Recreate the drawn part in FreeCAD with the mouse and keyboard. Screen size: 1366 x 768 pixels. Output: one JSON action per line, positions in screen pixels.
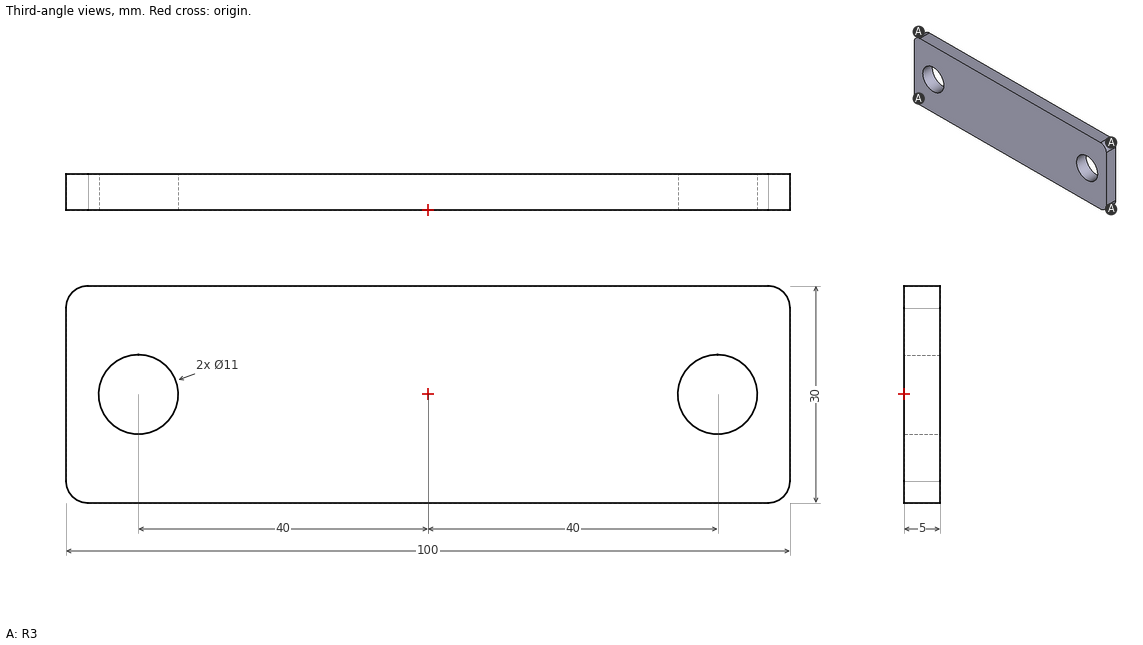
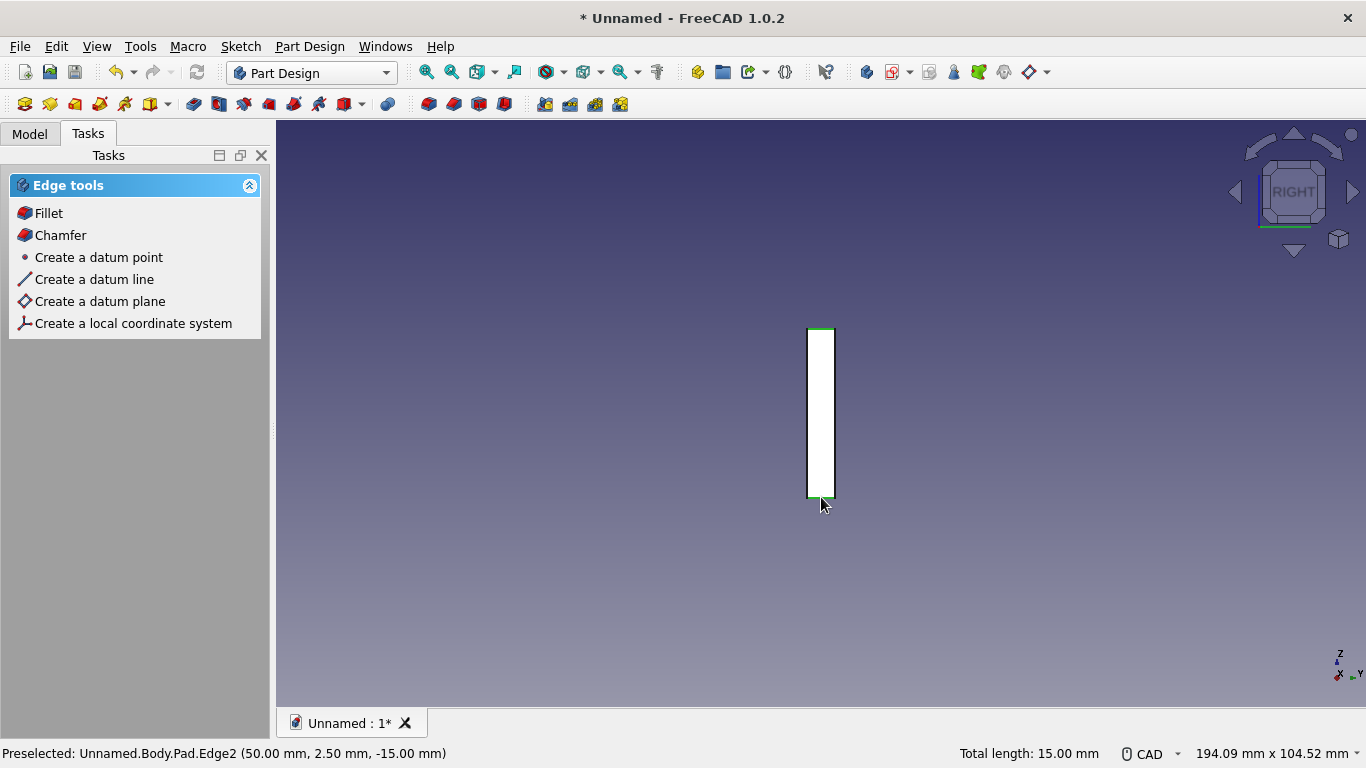
{"action": "key", "text": "5"}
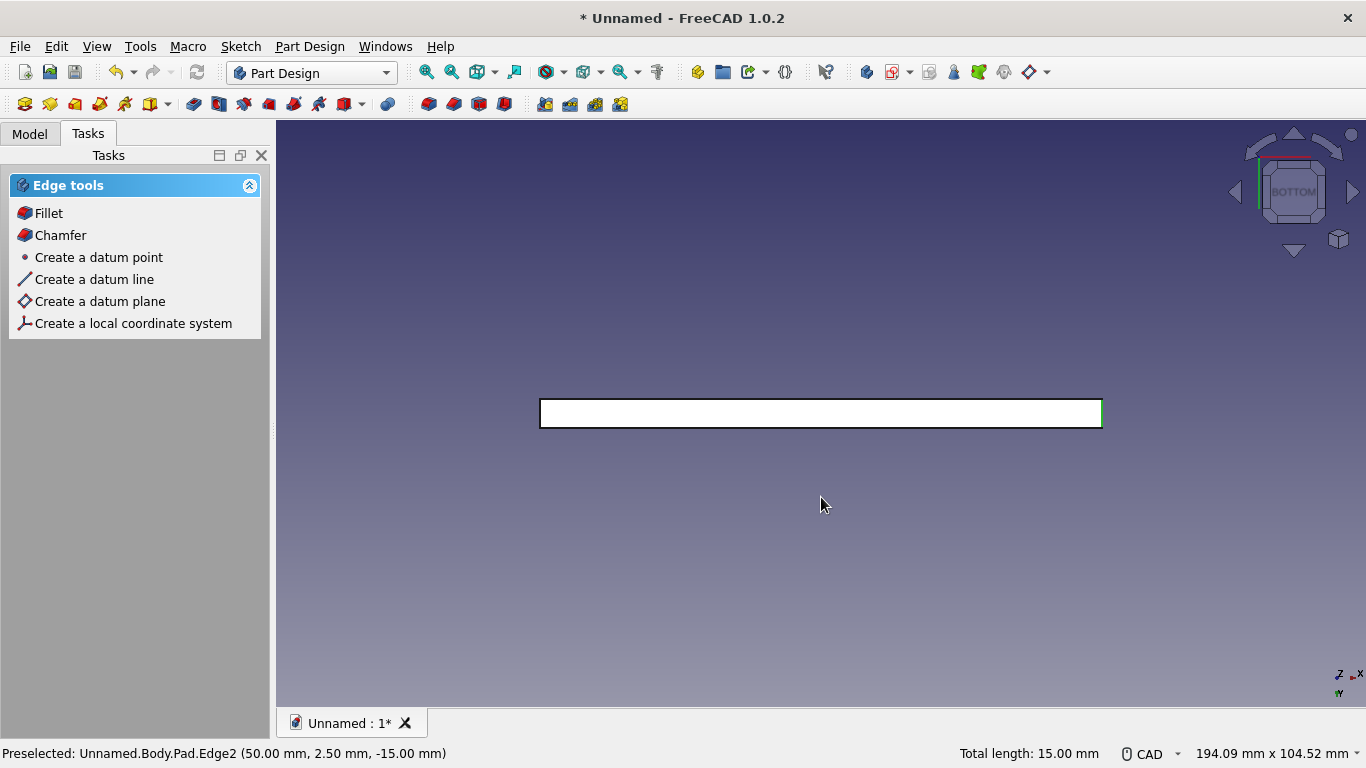
{"action": "left_click", "coordinate": [540, 412], "text": "ctrl"}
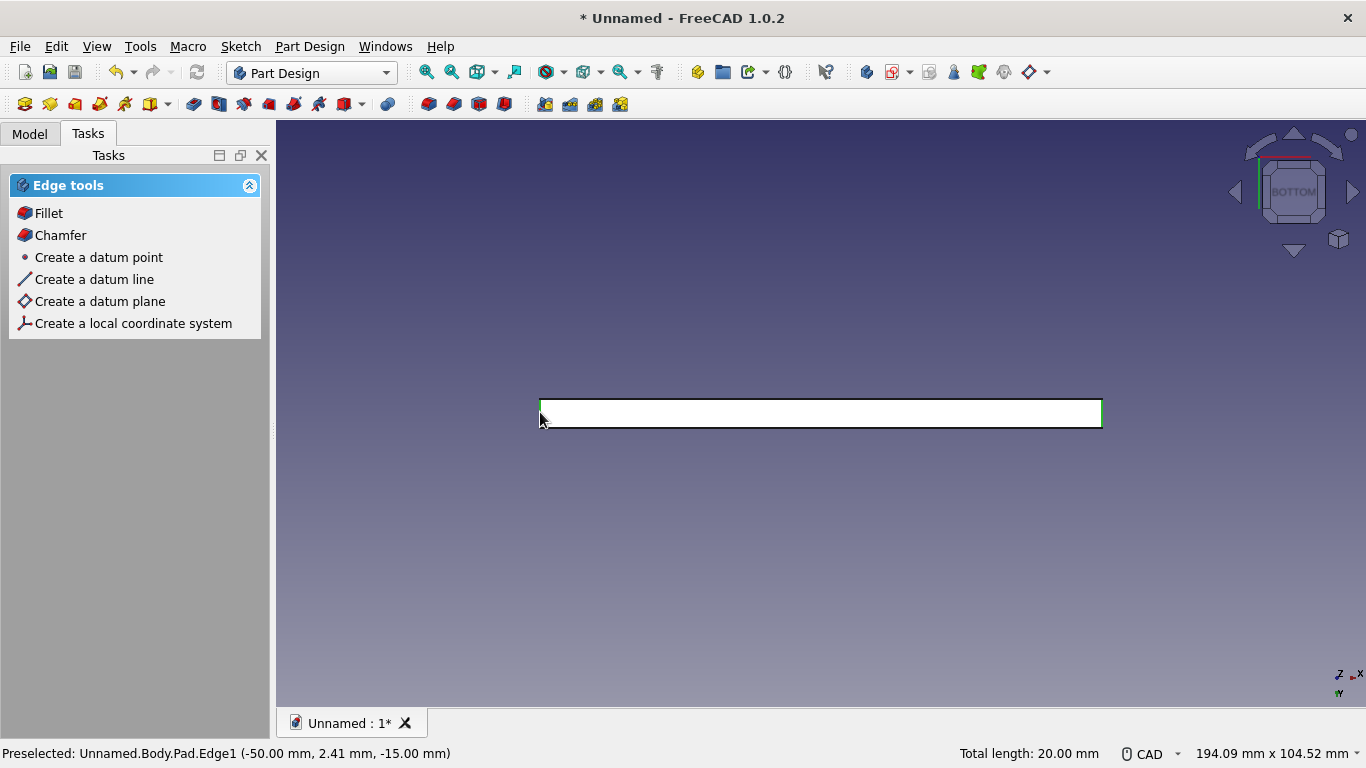
{"action": "left_click", "coordinate": [429, 104]}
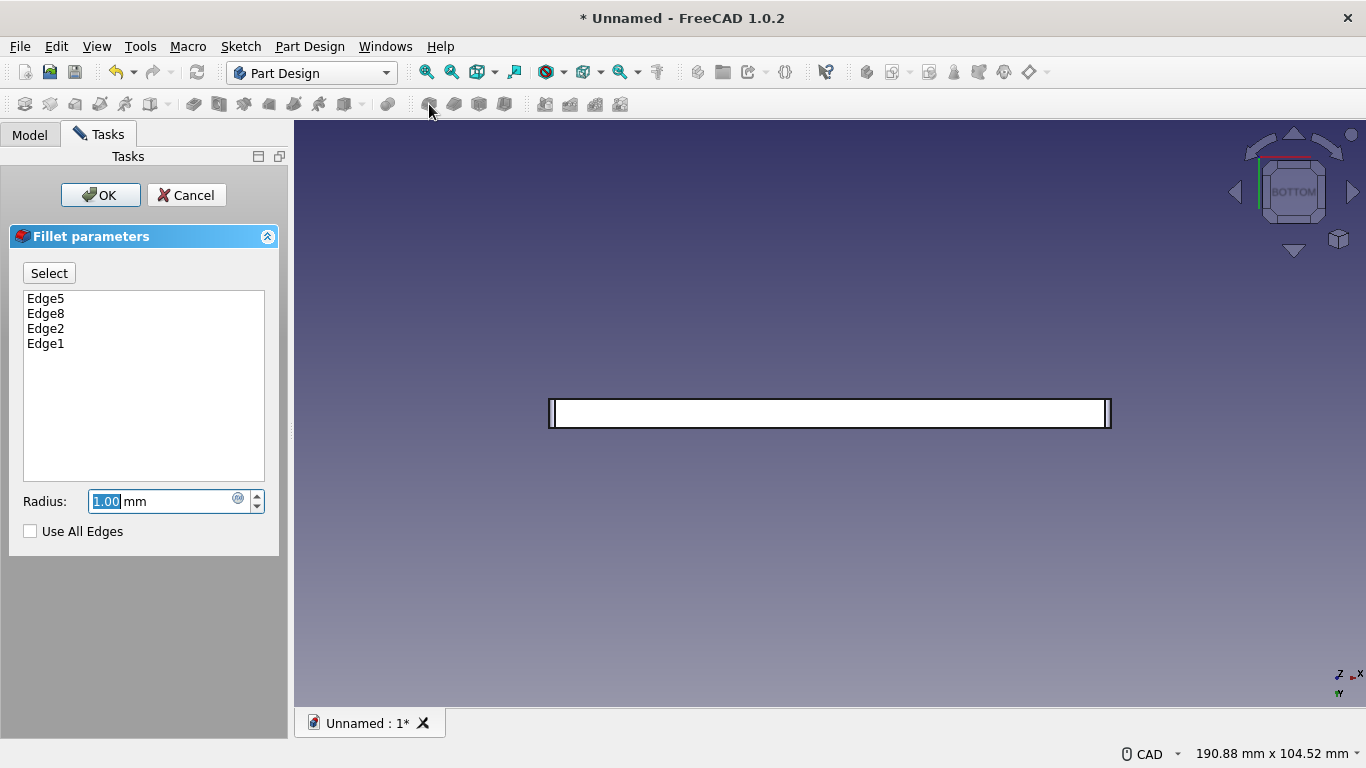
{"action": "type", "text": "3"}
{"action": "key", "text": "Tab"}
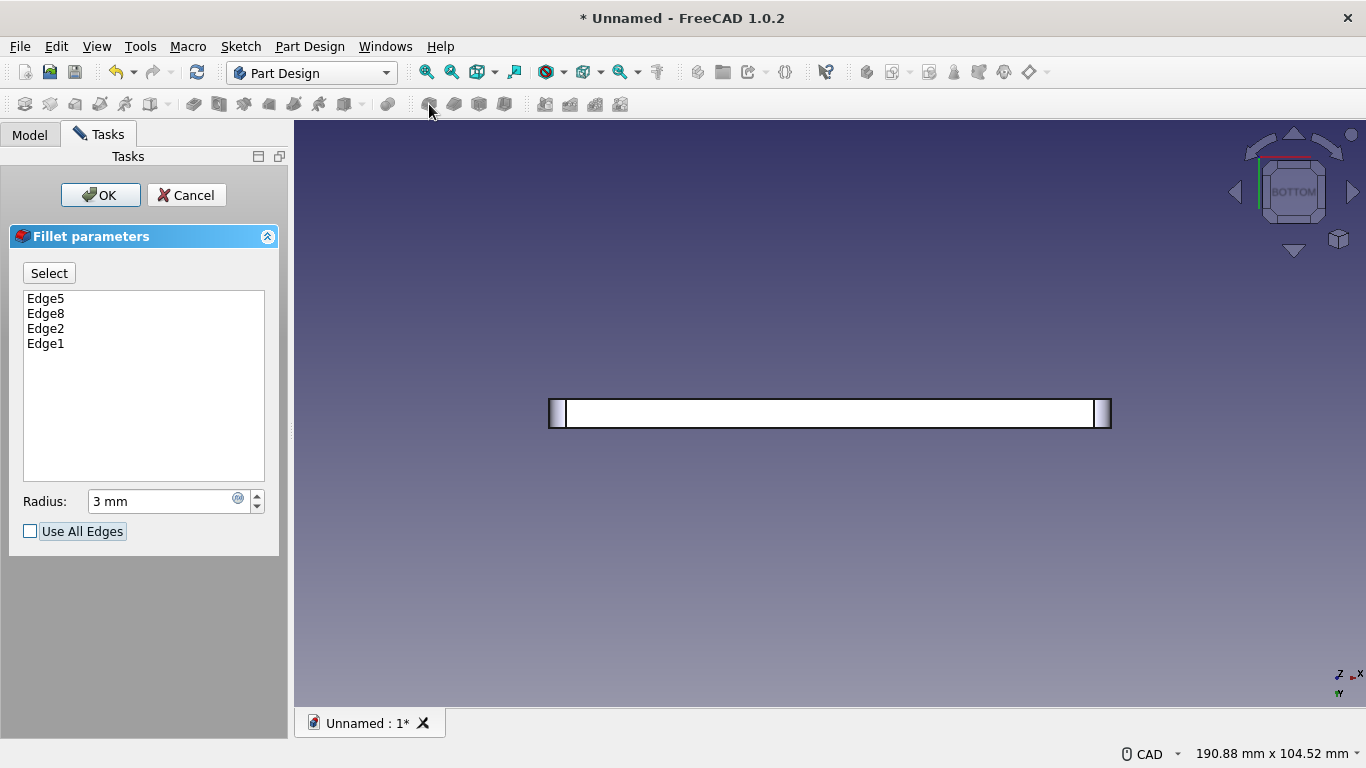
{"action": "left_click", "coordinate": [101, 195]}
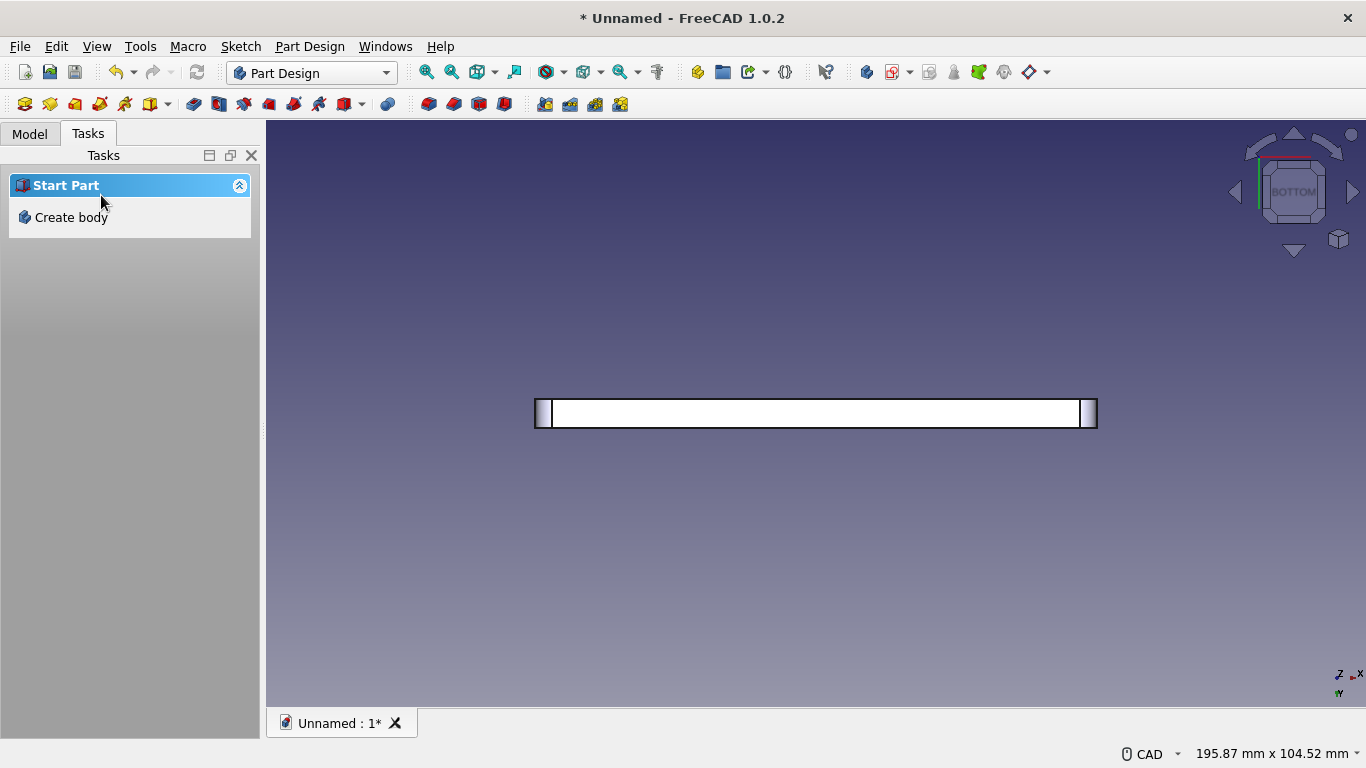
{"action": "key", "text": "4"}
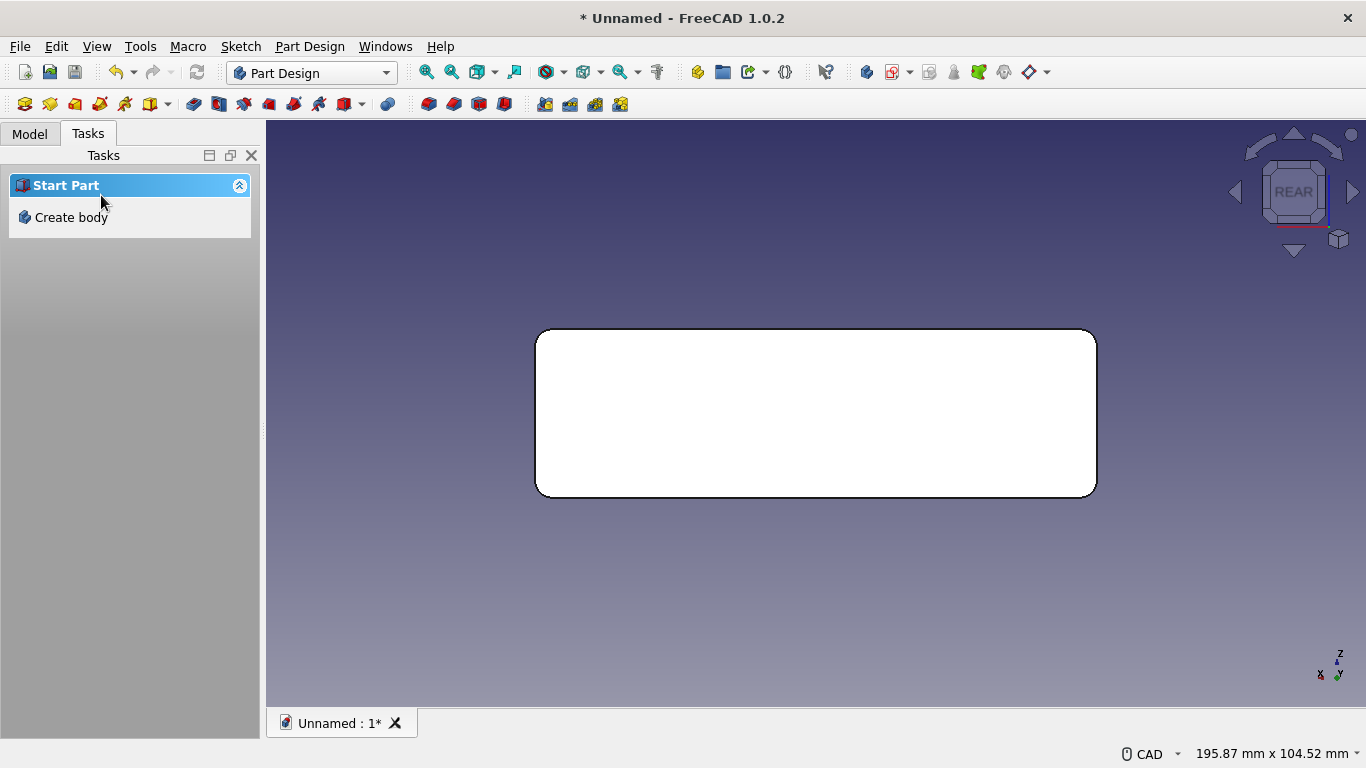
{"action": "left_click", "coordinate": [656, 412]}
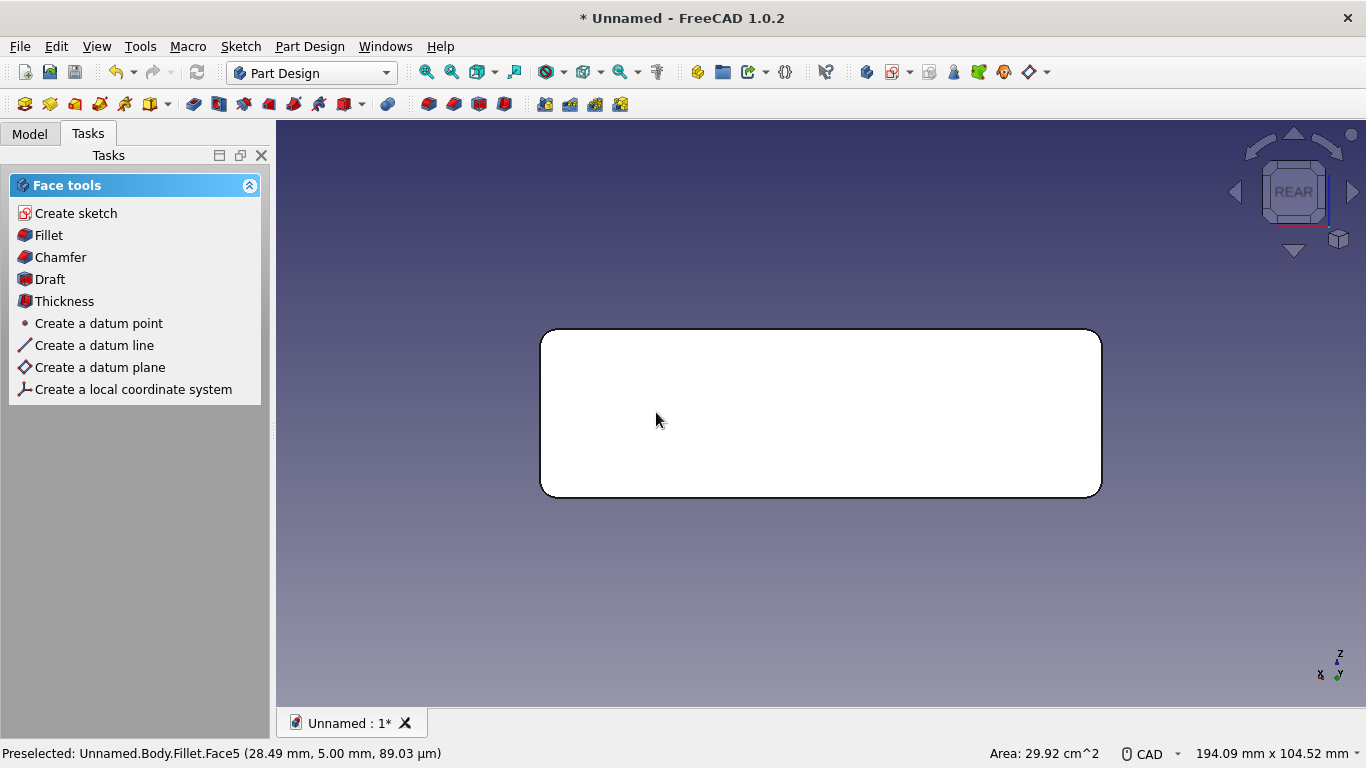
{"action": "left_click", "coordinate": [892, 72]}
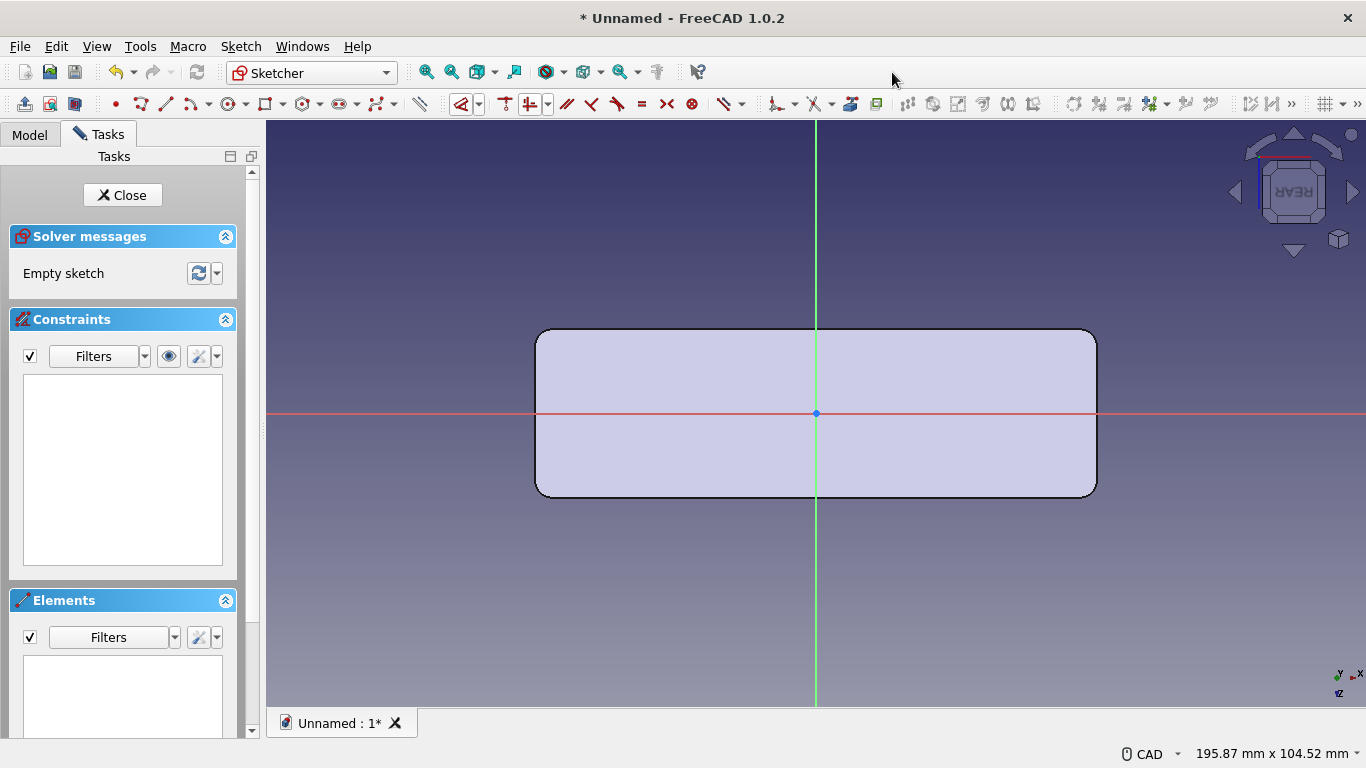
{"action": "key", "text": "g c"}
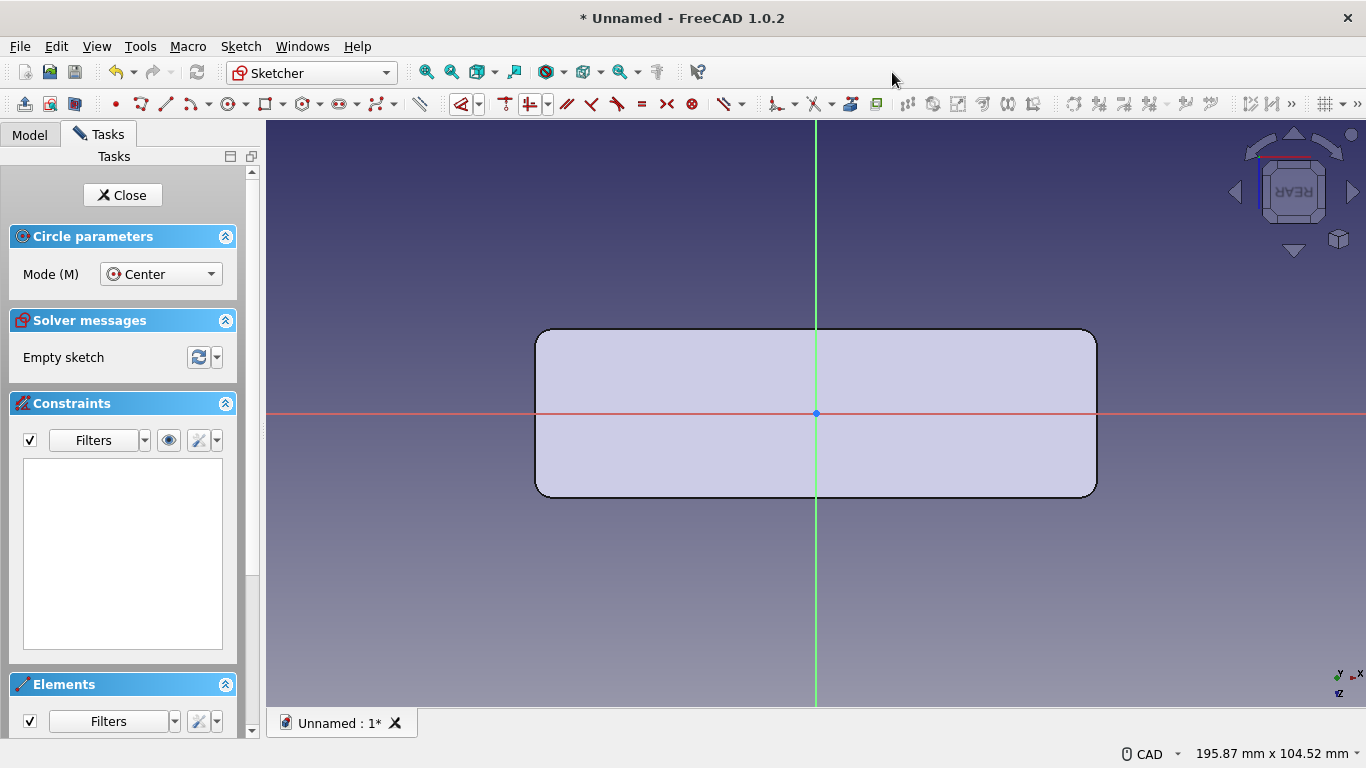
{"action": "left_click", "coordinate": [591, 414]}
{"action": "mouse_move", "coordinate": [613, 392]}